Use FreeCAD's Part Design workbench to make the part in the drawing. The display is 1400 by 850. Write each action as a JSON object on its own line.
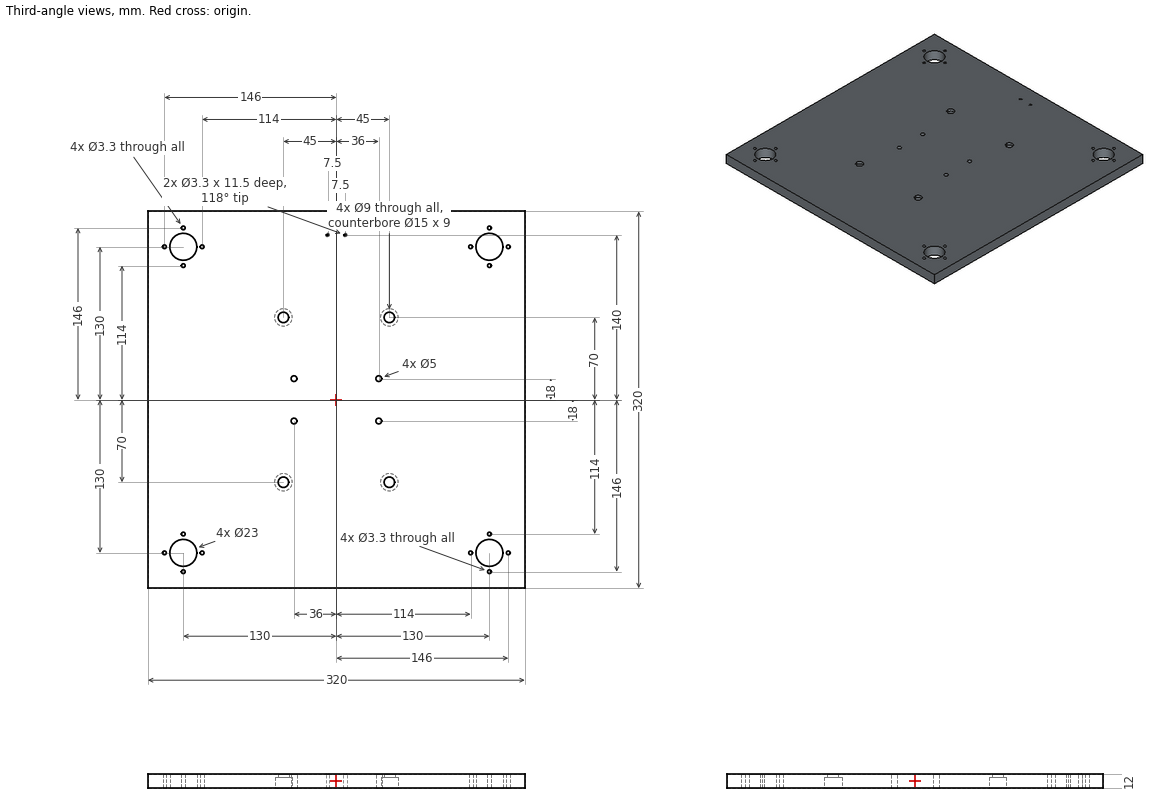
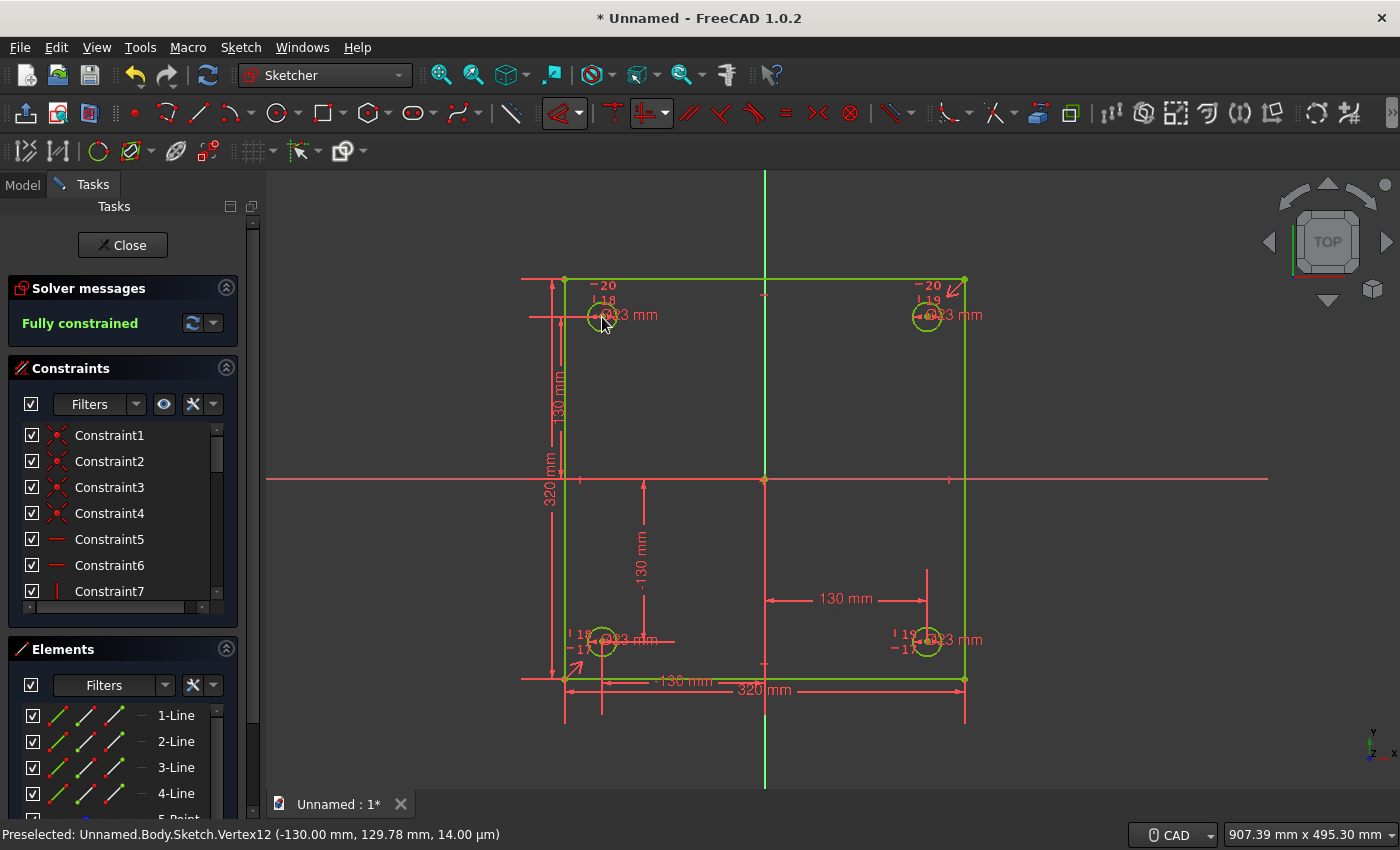
{"action": "left_click", "coordinate": [123, 245]}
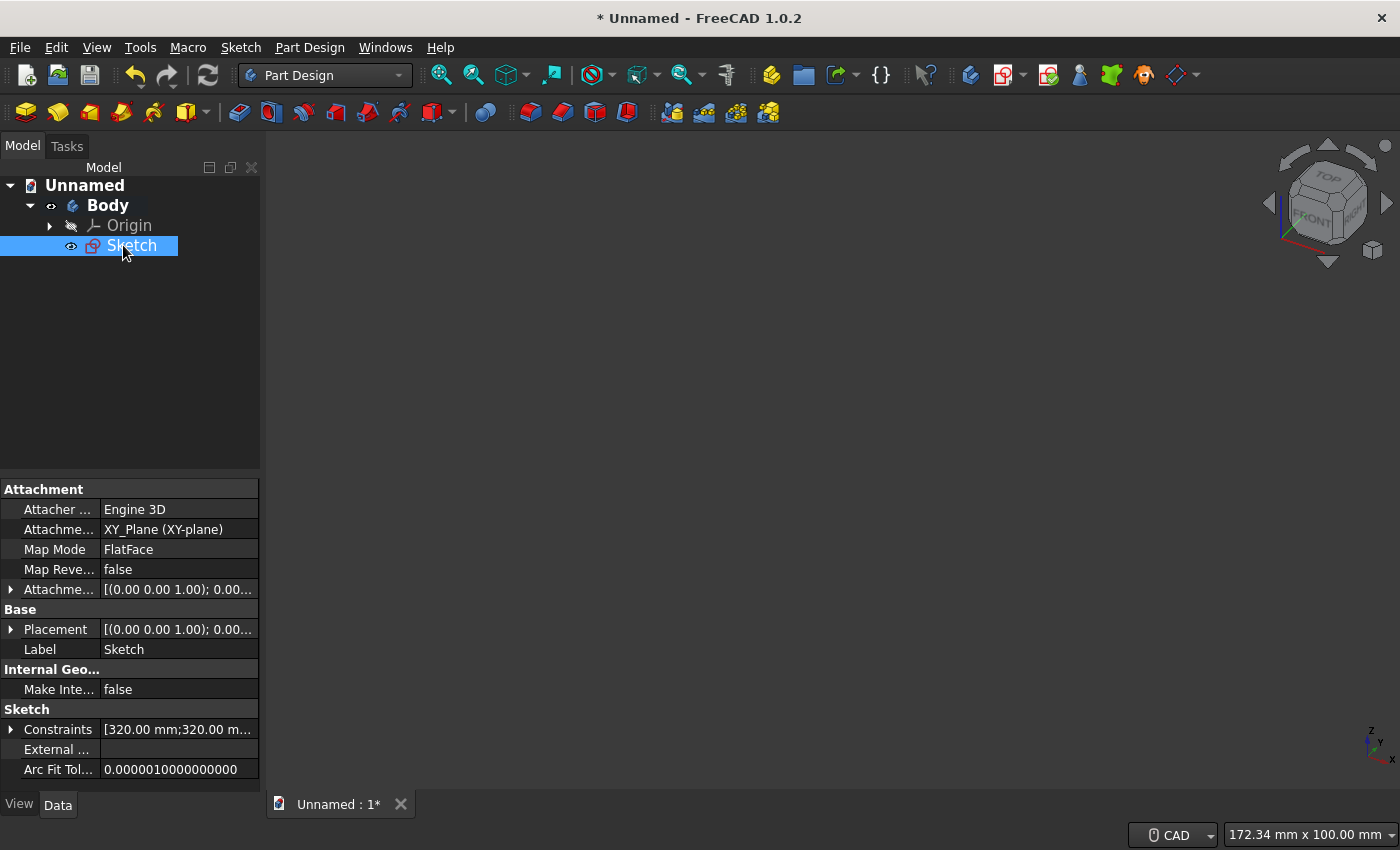
{"action": "left_click", "coordinate": [26, 112]}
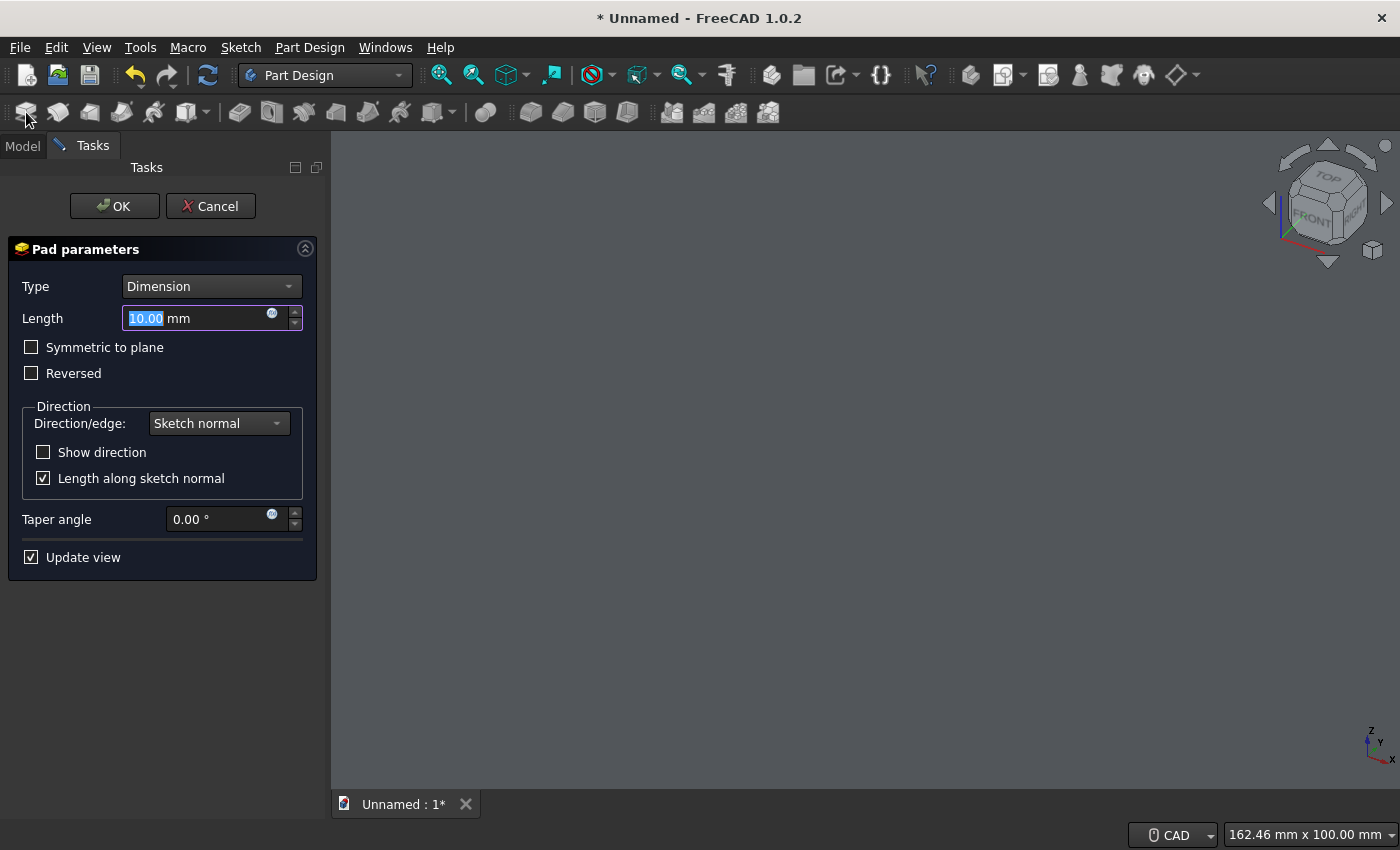
{"action": "type", "text": "12"}
{"action": "key", "text": "Tab"}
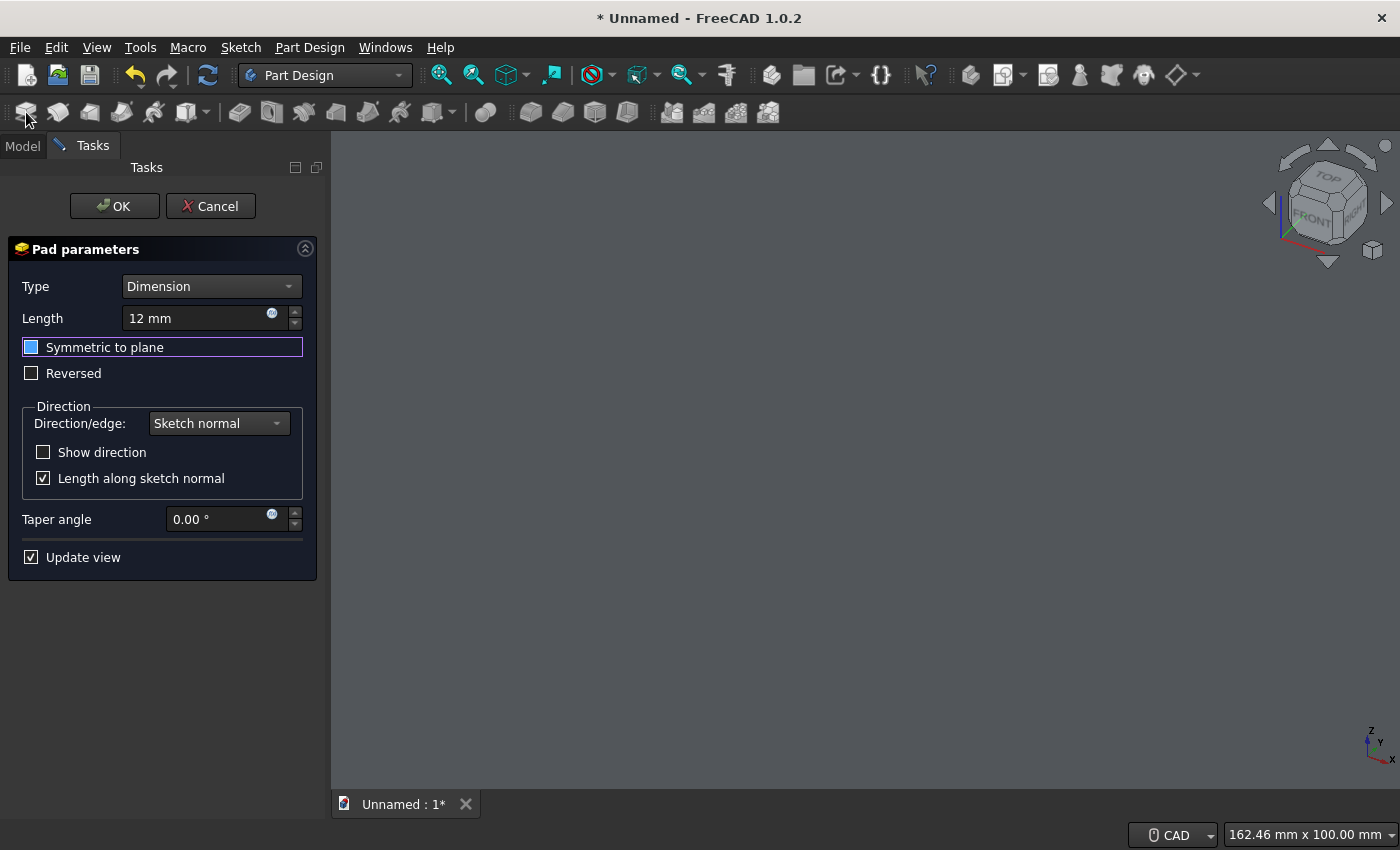
{"action": "left_click", "coordinate": [30, 347]}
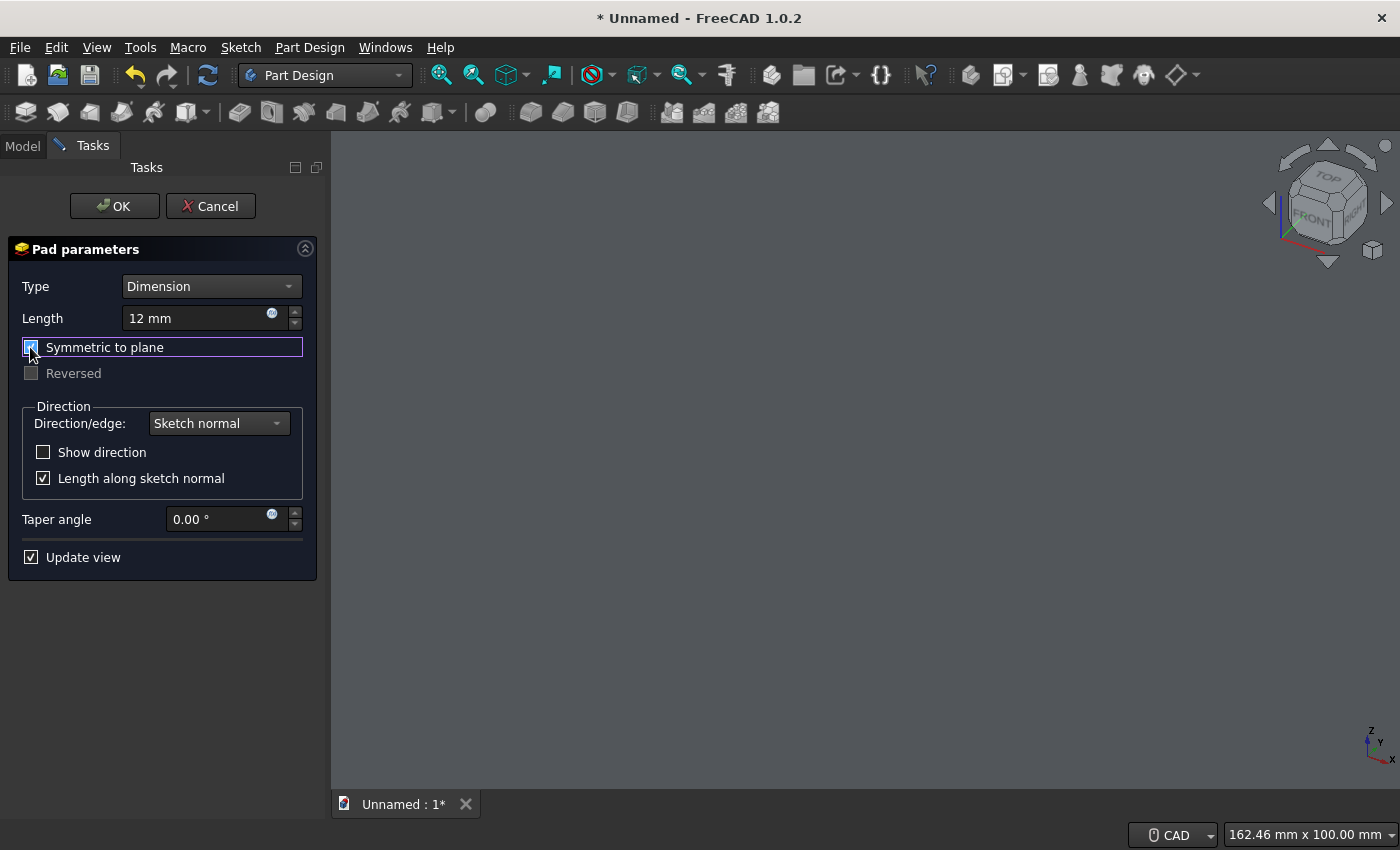
{"action": "left_click", "coordinate": [115, 206]}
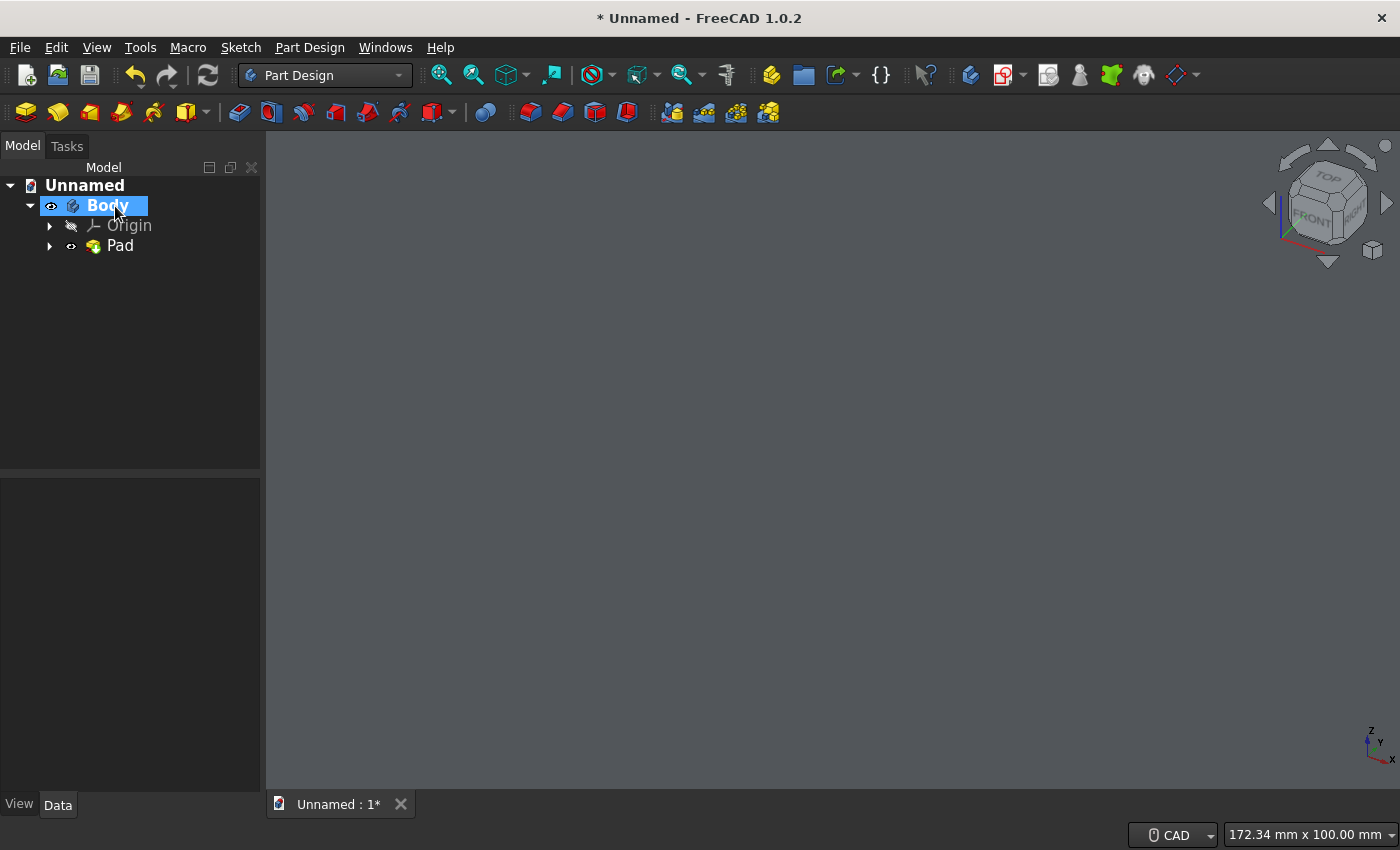
{"action": "left_click", "coordinate": [442, 76]}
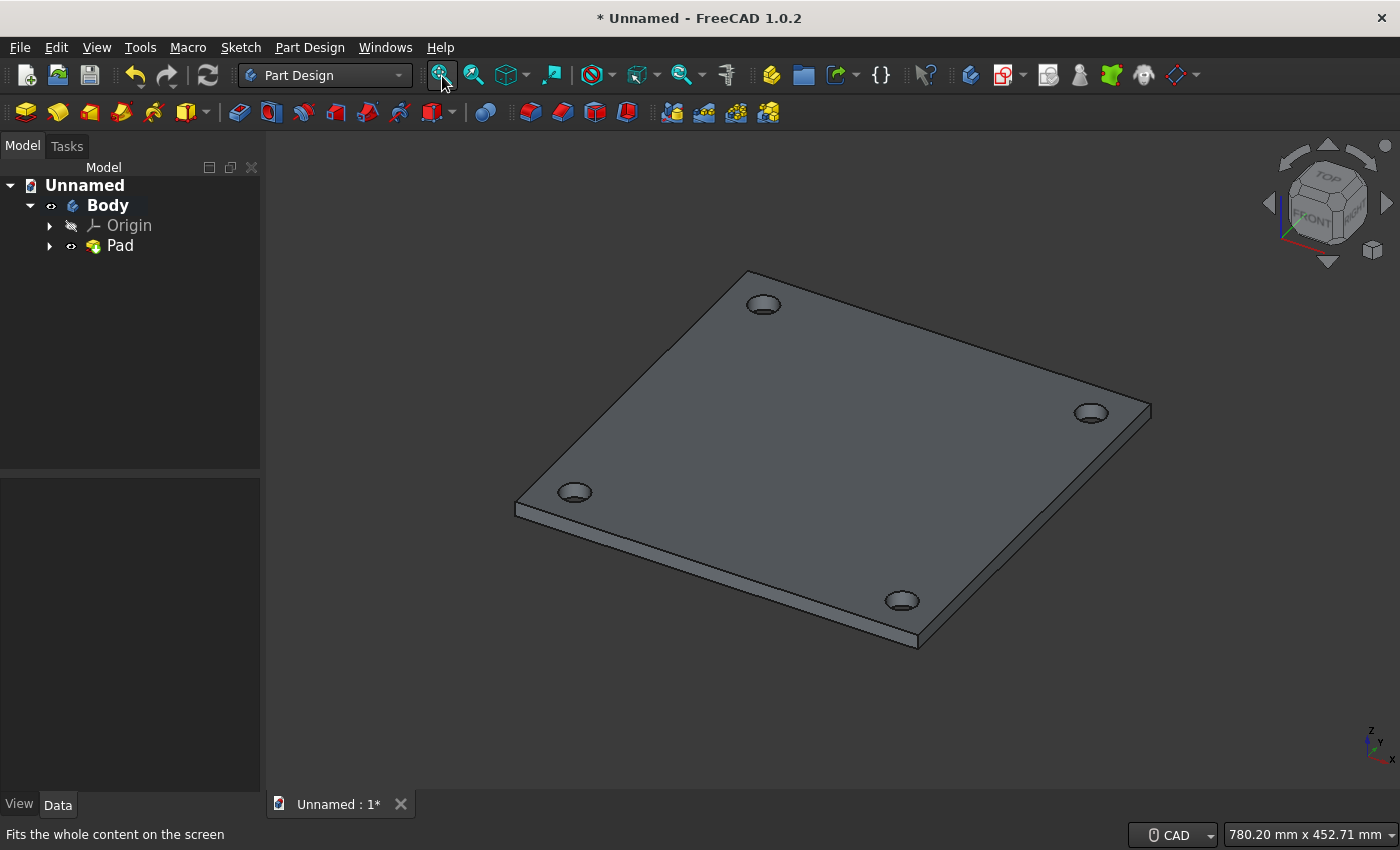
{"action": "key", "text": "5"}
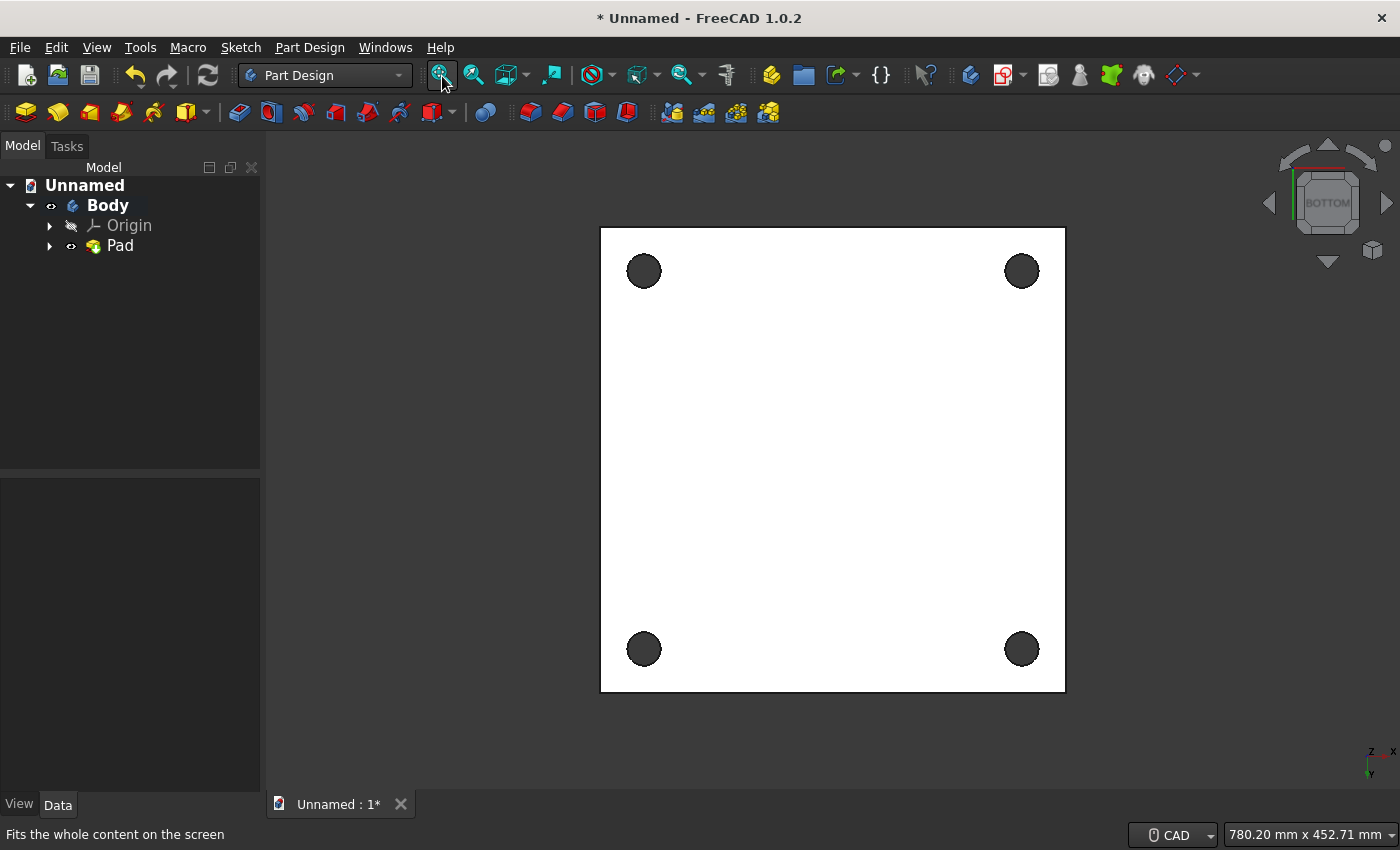
{"action": "left_click", "coordinate": [833, 459]}